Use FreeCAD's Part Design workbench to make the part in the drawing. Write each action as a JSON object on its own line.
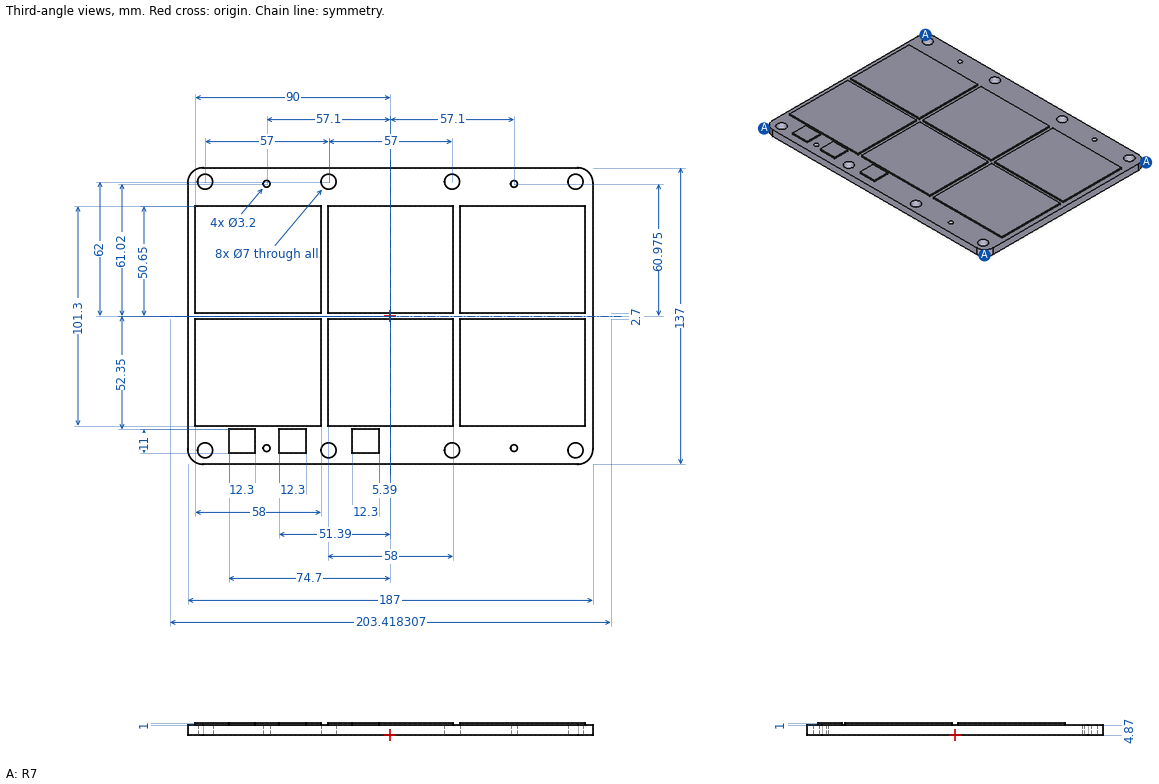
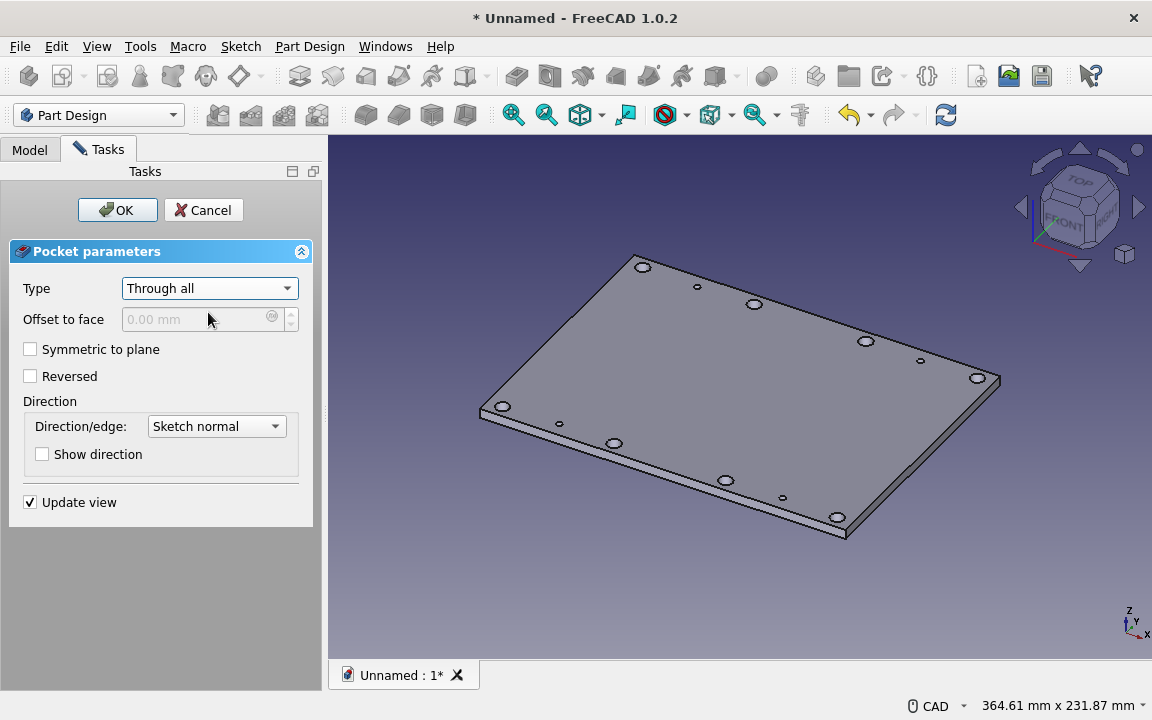
{"action": "left_click", "coordinate": [118, 210]}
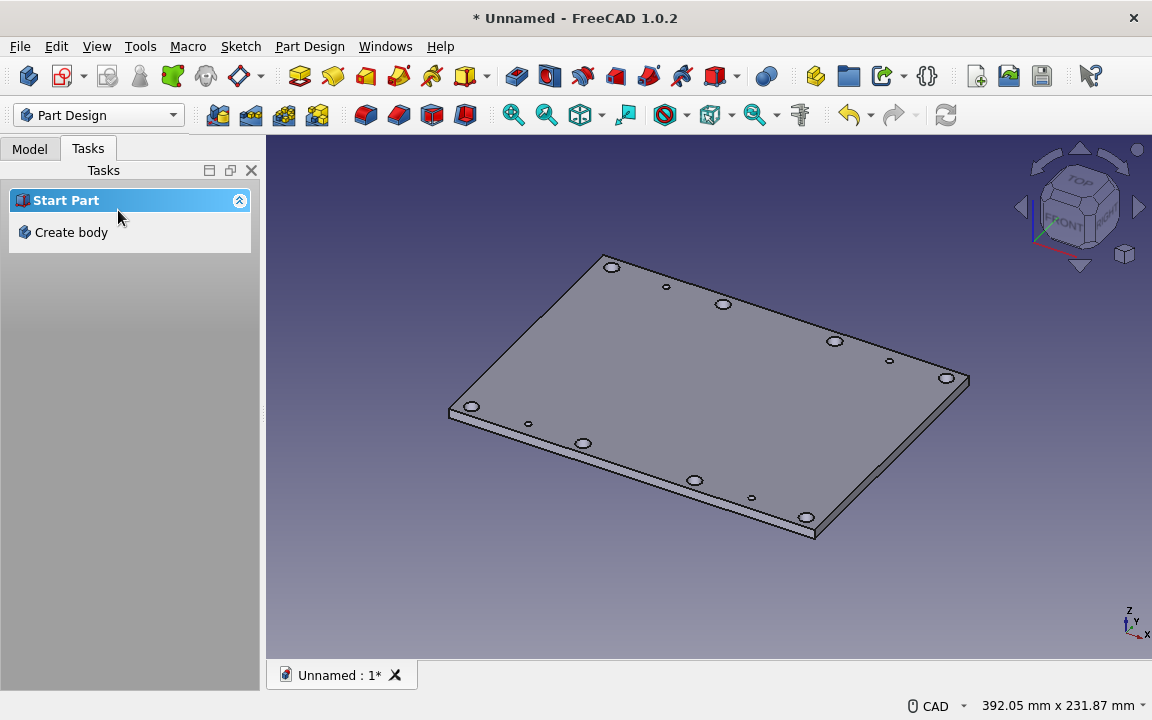
{"action": "left_click", "coordinate": [709, 391]}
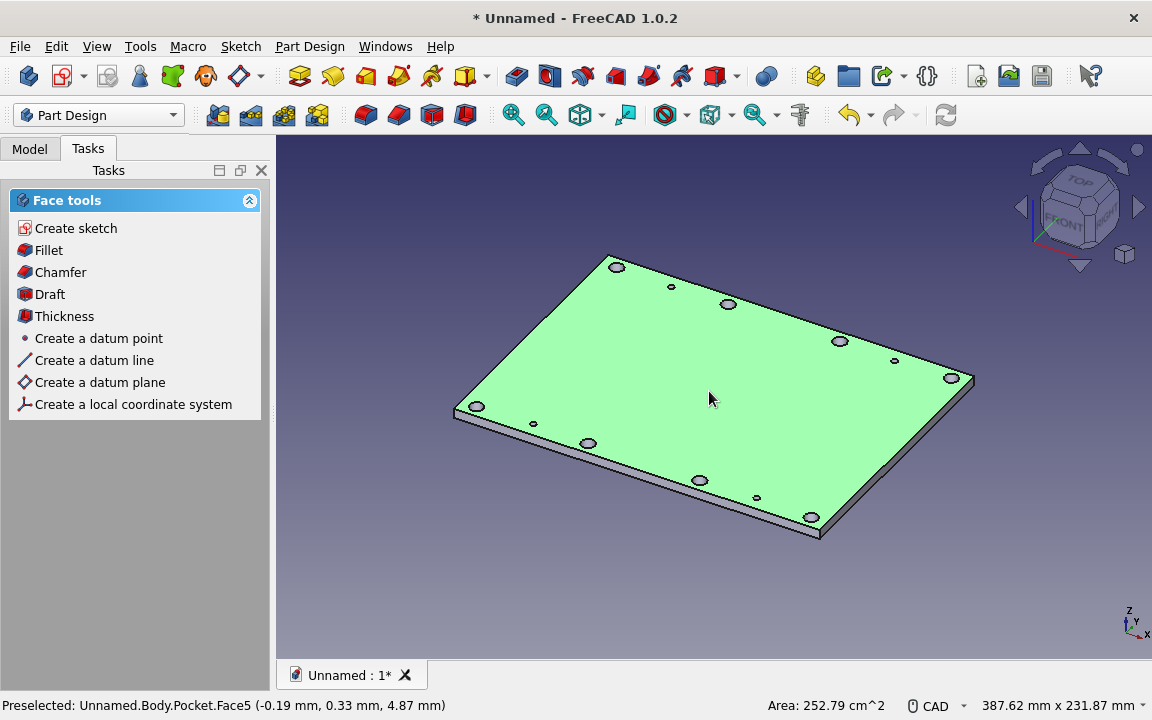
{"action": "left_click", "coordinate": [62, 76]}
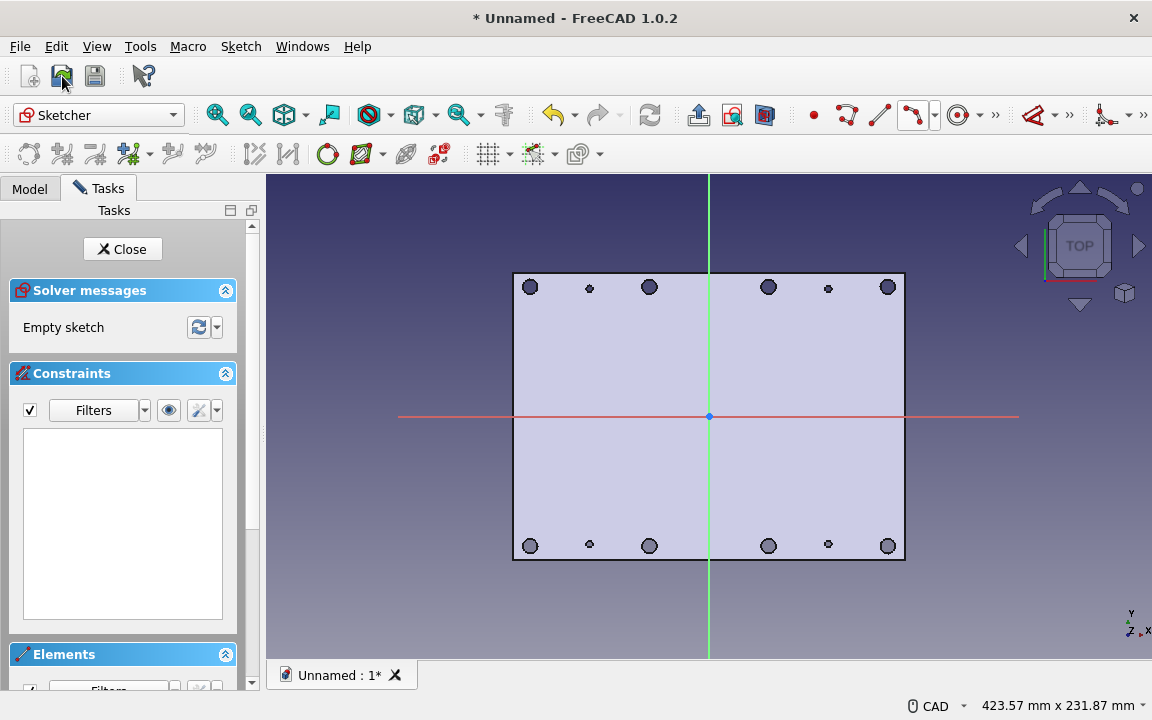
{"action": "key", "text": "g r"}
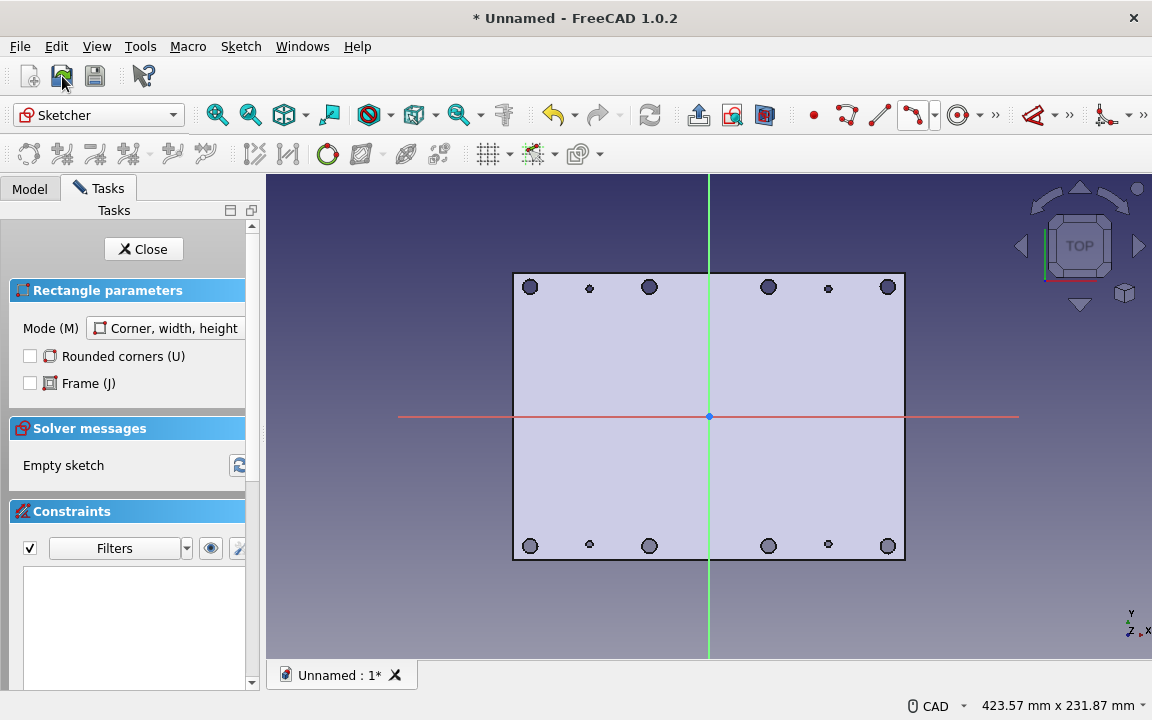
{"action": "left_click", "coordinate": [521, 311]}
{"action": "left_click", "coordinate": [642, 522]}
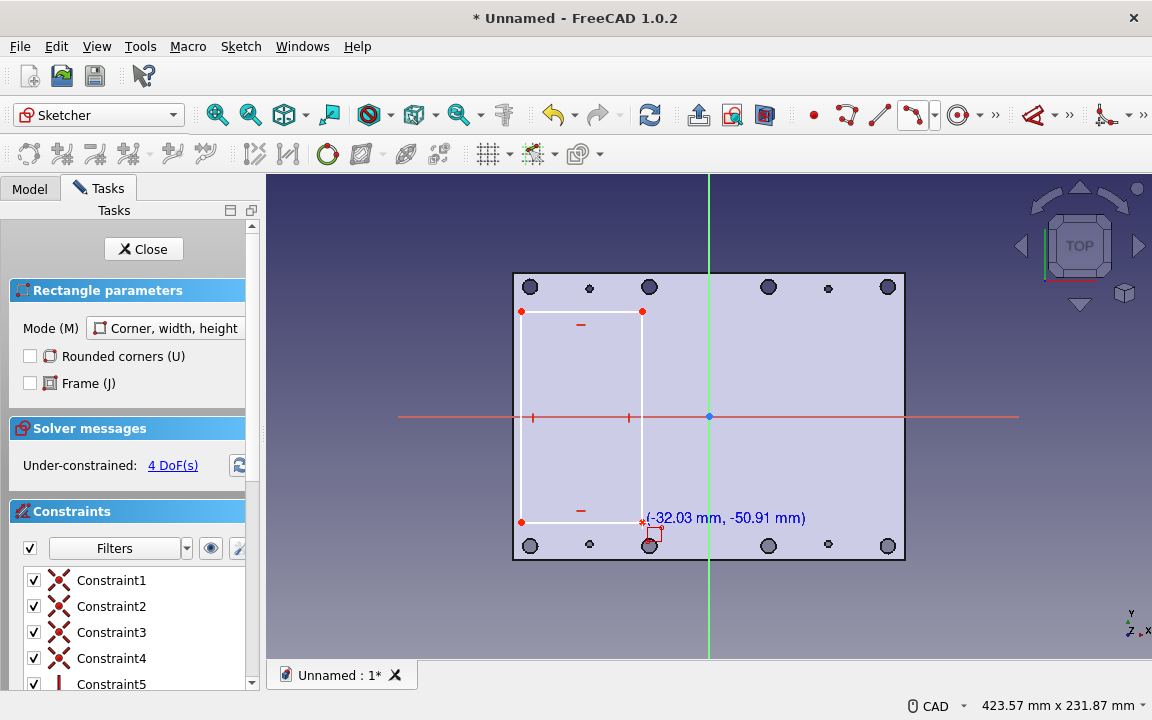
{"action": "key", "text": "g v"}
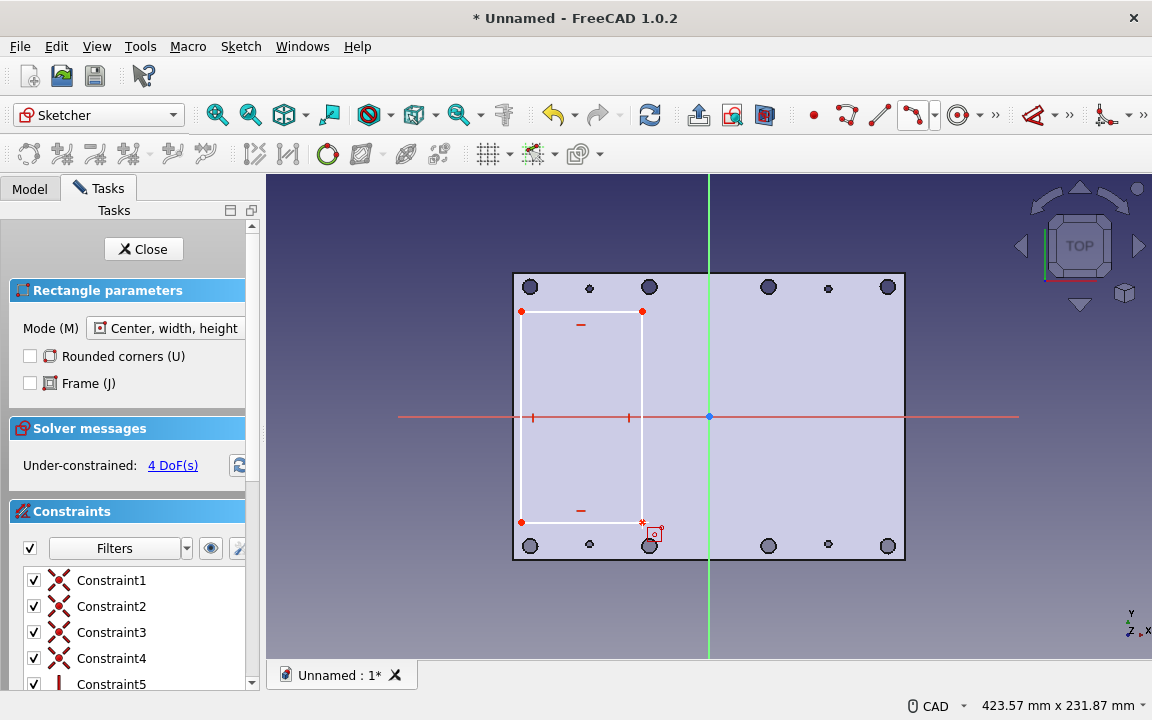
{"action": "left_click", "coordinate": [709, 416]}
{"action": "left_click", "coordinate": [770, 311]}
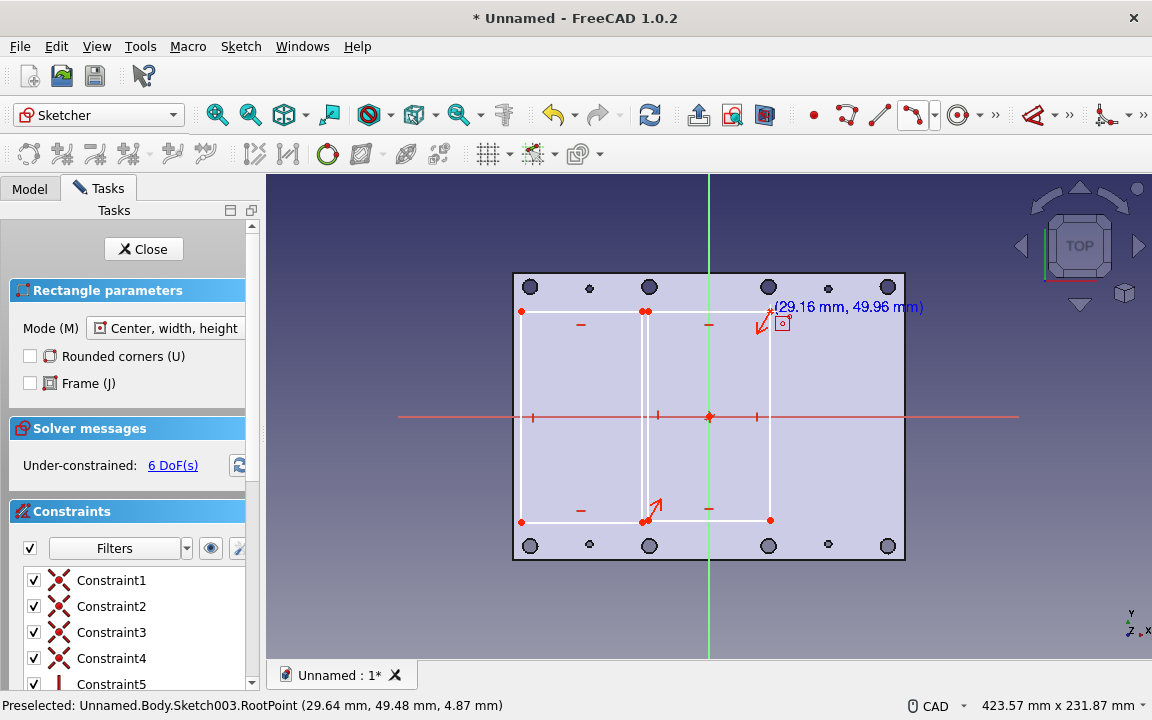
{"action": "key", "text": "g r"}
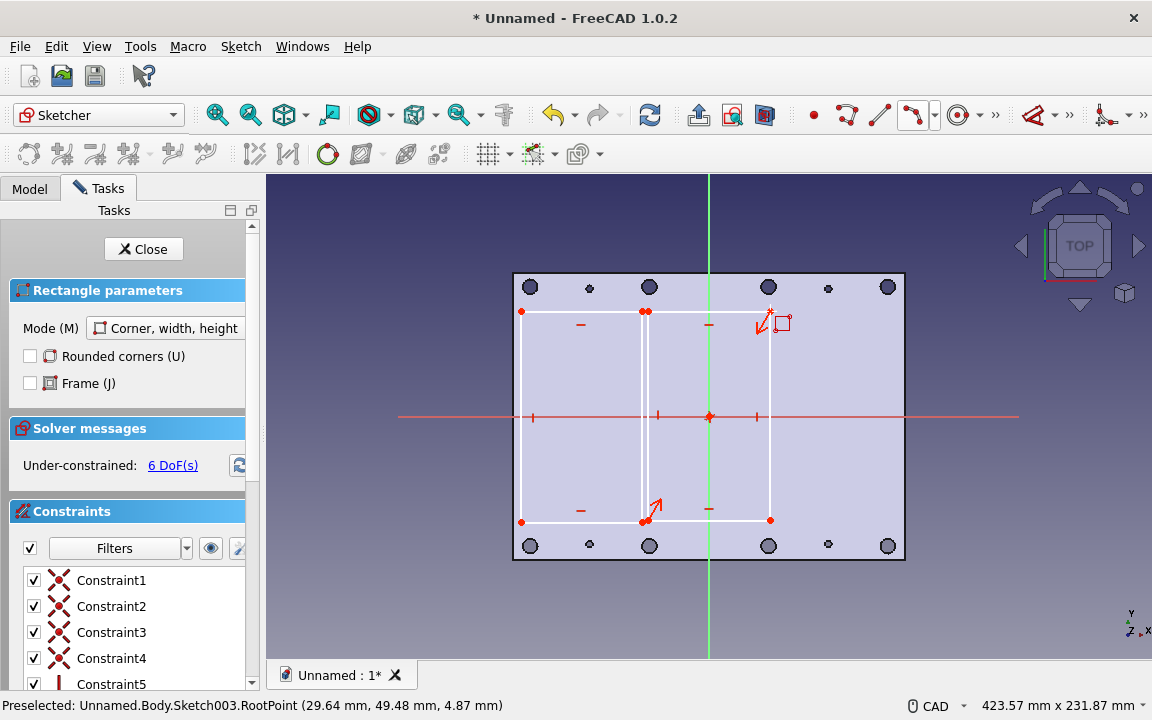
{"action": "scroll", "coordinate": [776, 311], "scroll_direction": "up", "scroll_amount": 5}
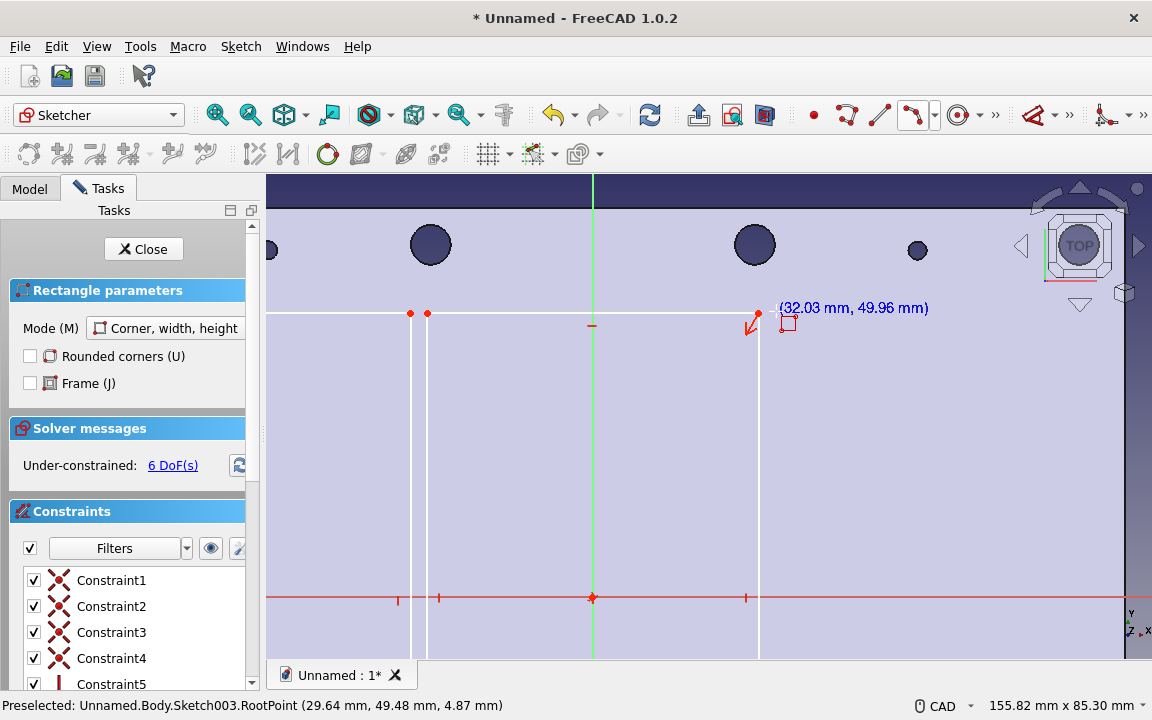
{"action": "left_click", "coordinate": [775, 309]}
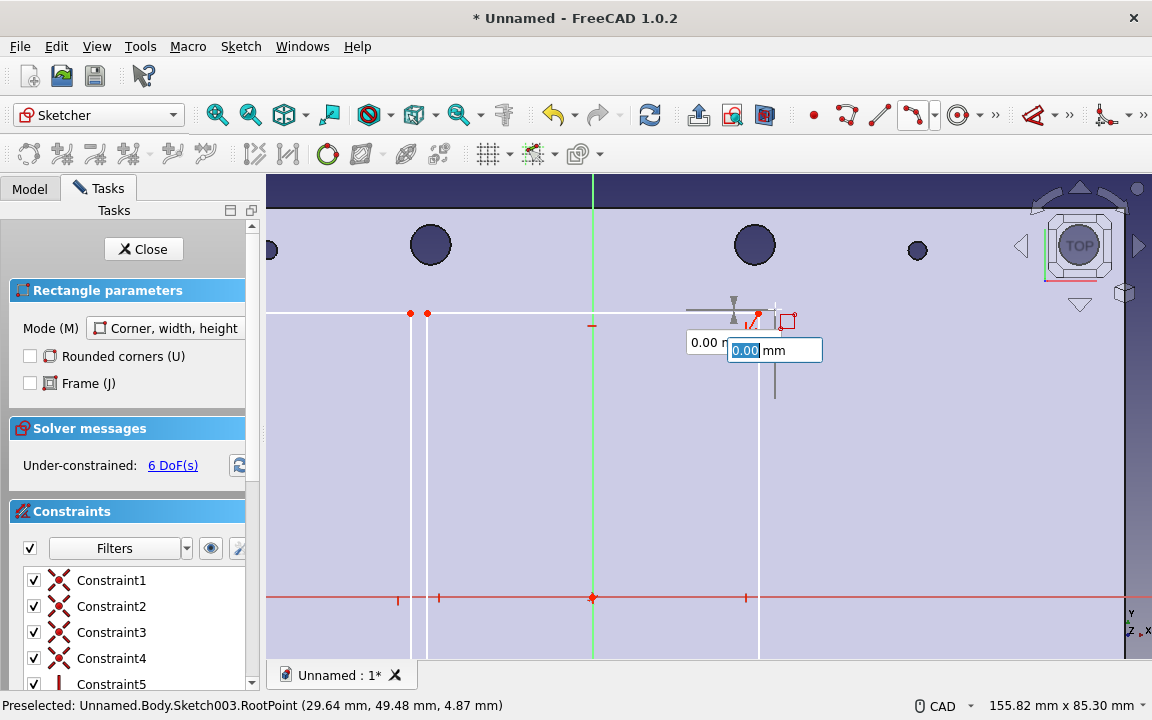
{"action": "scroll", "coordinate": [679, 269], "scroll_direction": "down", "scroll_amount": 4}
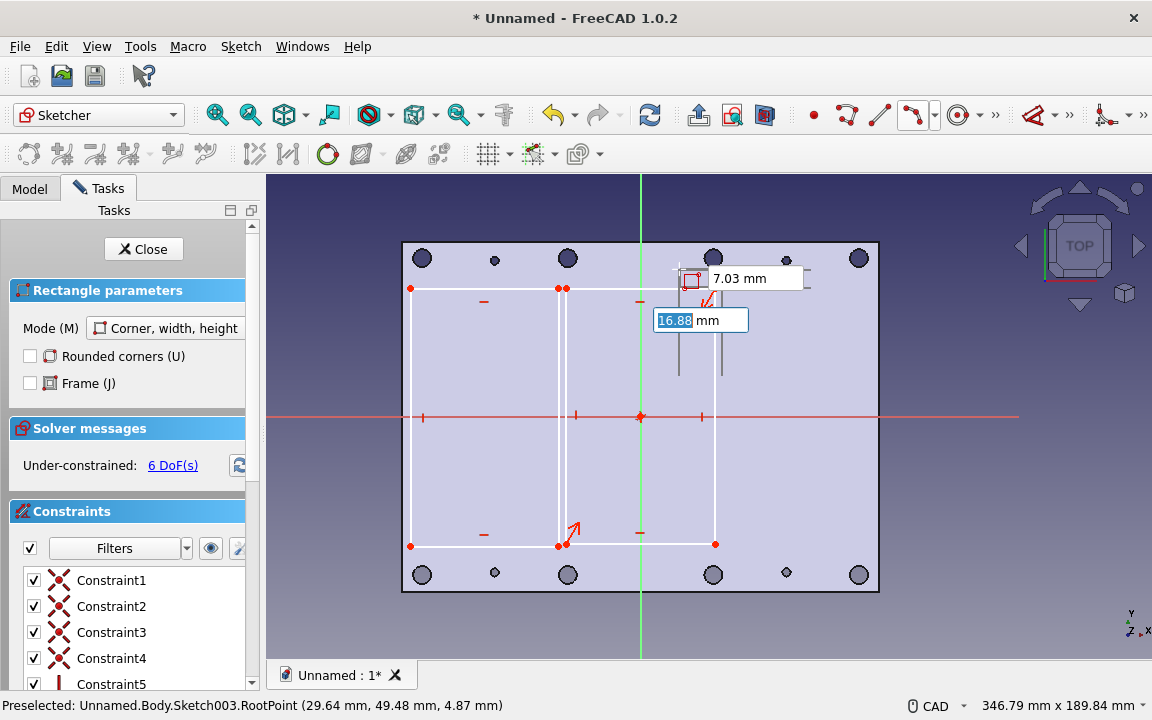
{"action": "left_click", "coordinate": [870, 546]}
{"action": "key", "text": "Escape"}